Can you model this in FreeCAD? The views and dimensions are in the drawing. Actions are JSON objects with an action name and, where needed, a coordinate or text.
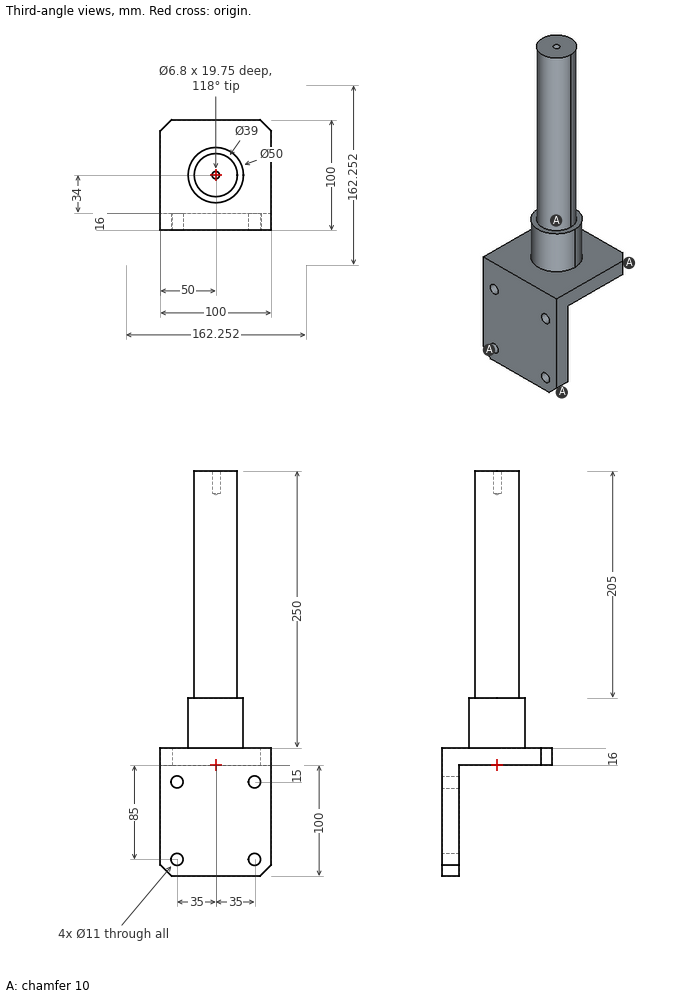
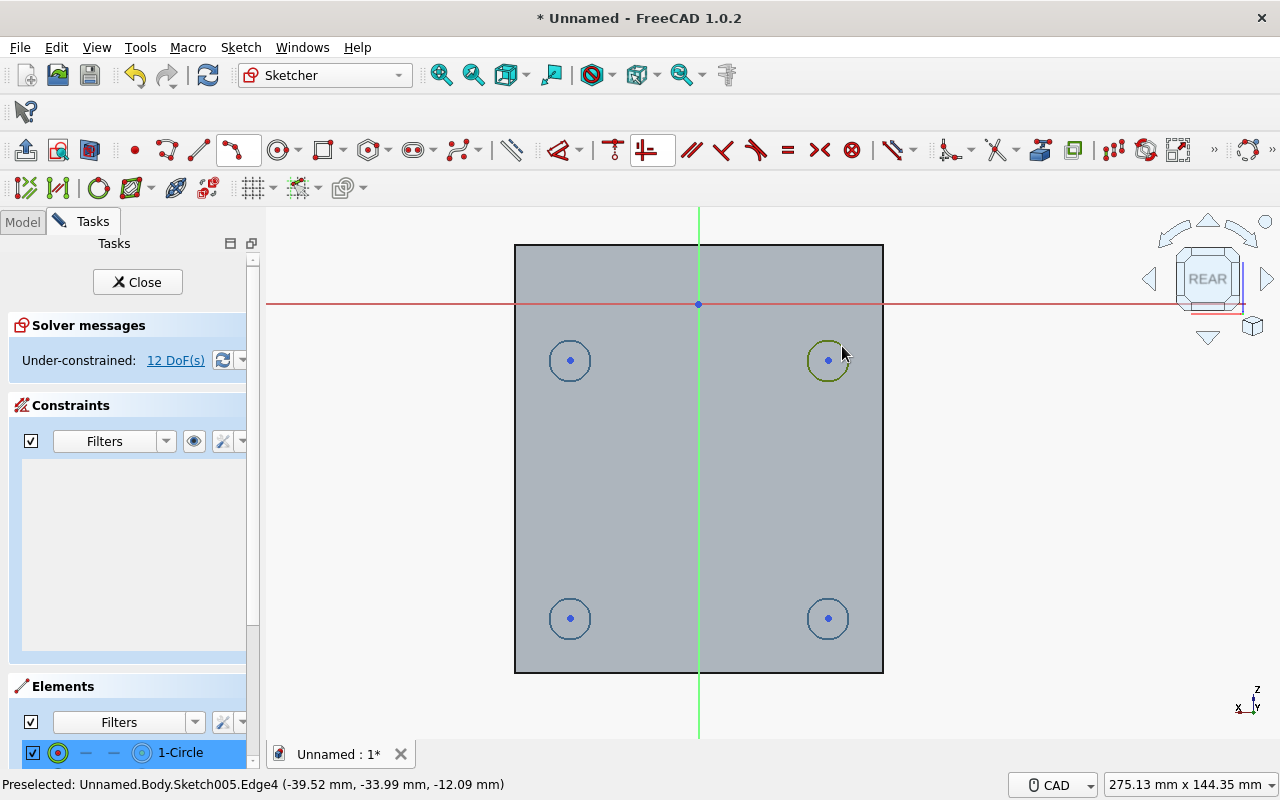
{"action": "key", "text": "e"}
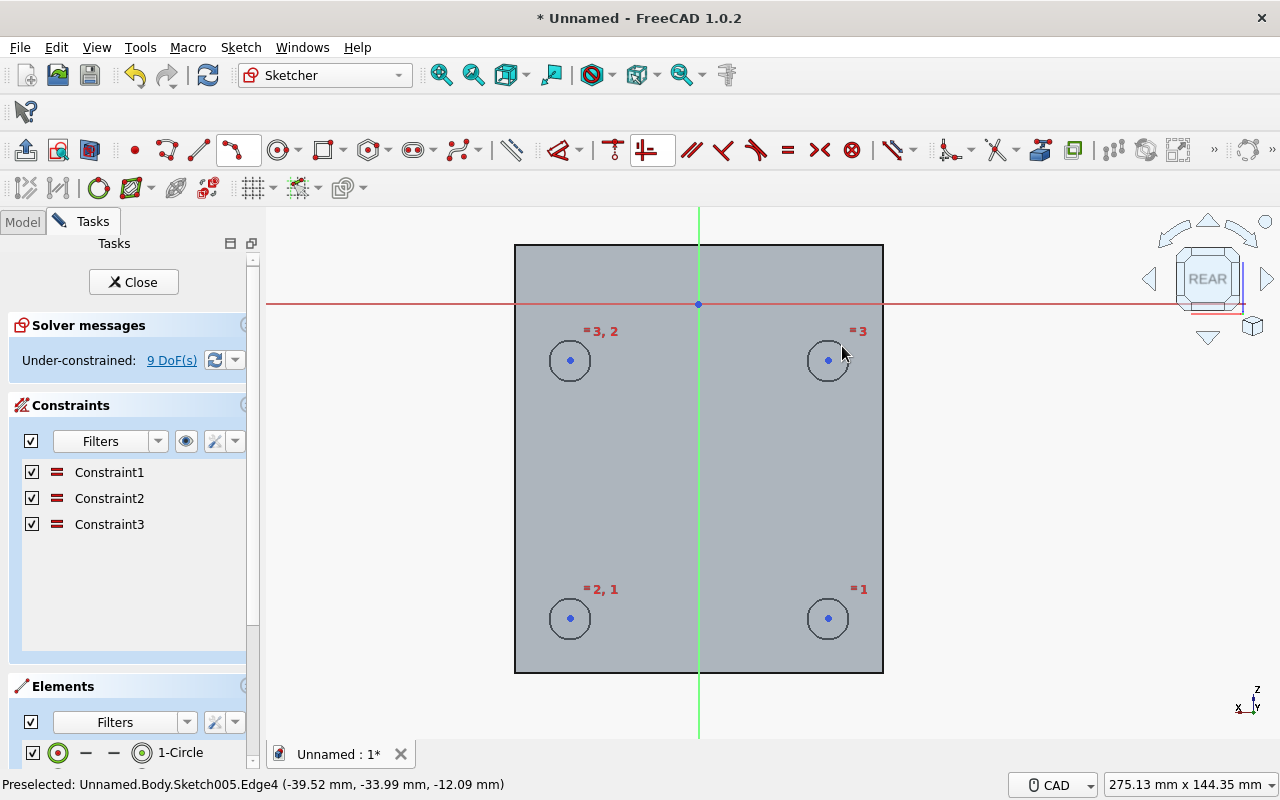
{"action": "left_click", "coordinate": [828, 619]}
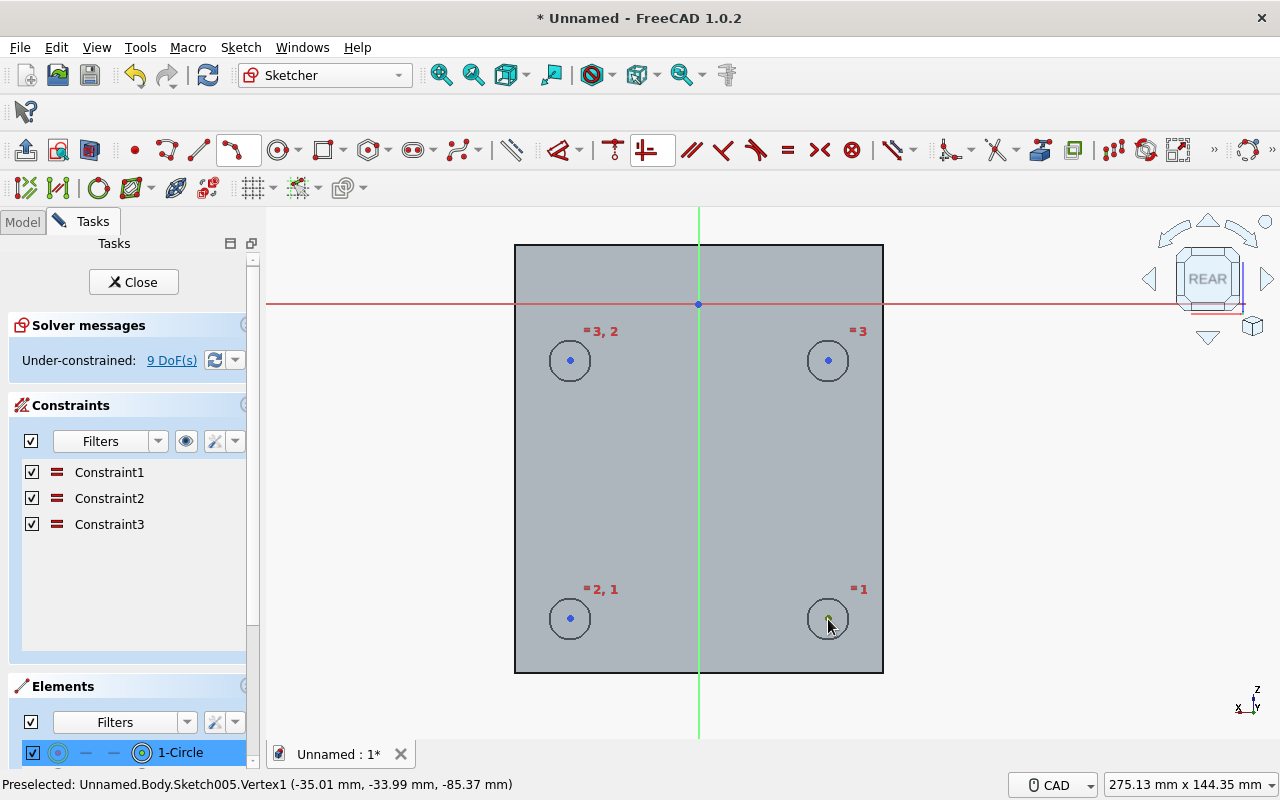
{"action": "left_click", "coordinate": [570, 619]}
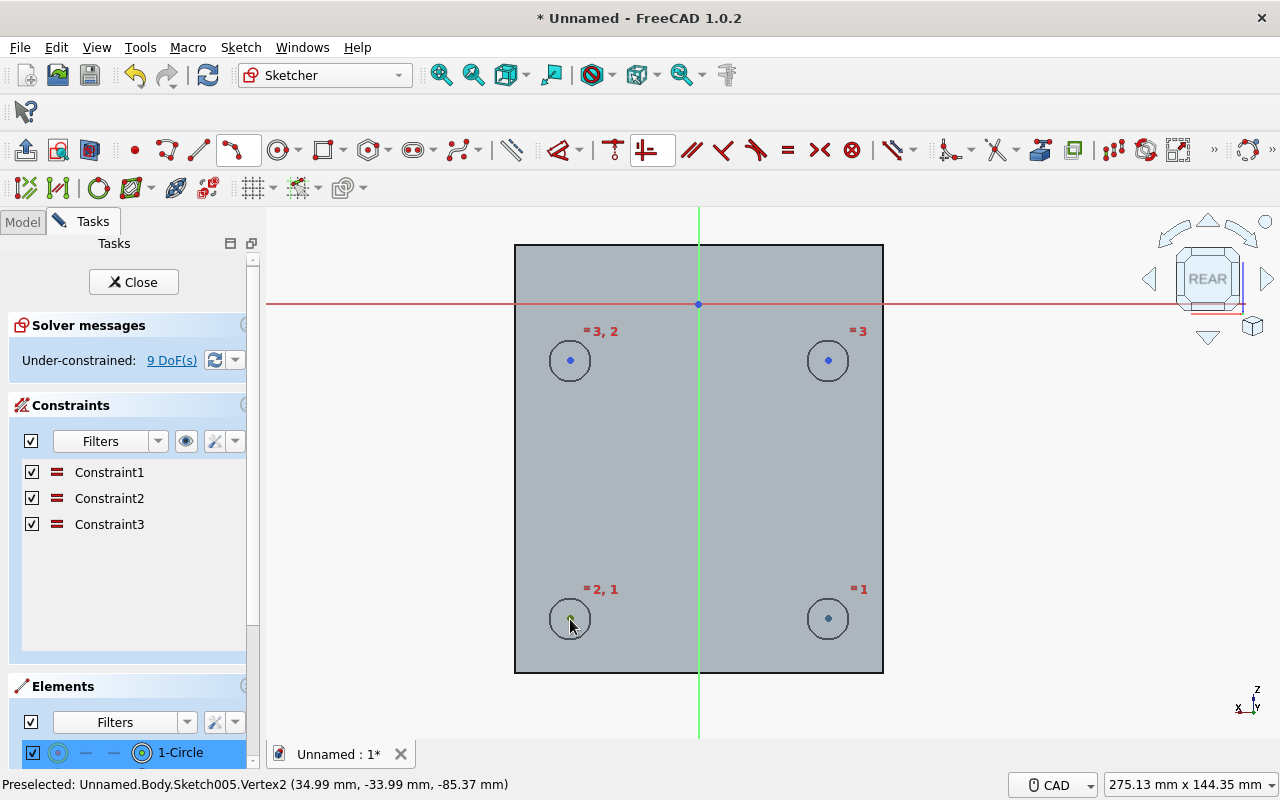
{"action": "key", "text": "h"}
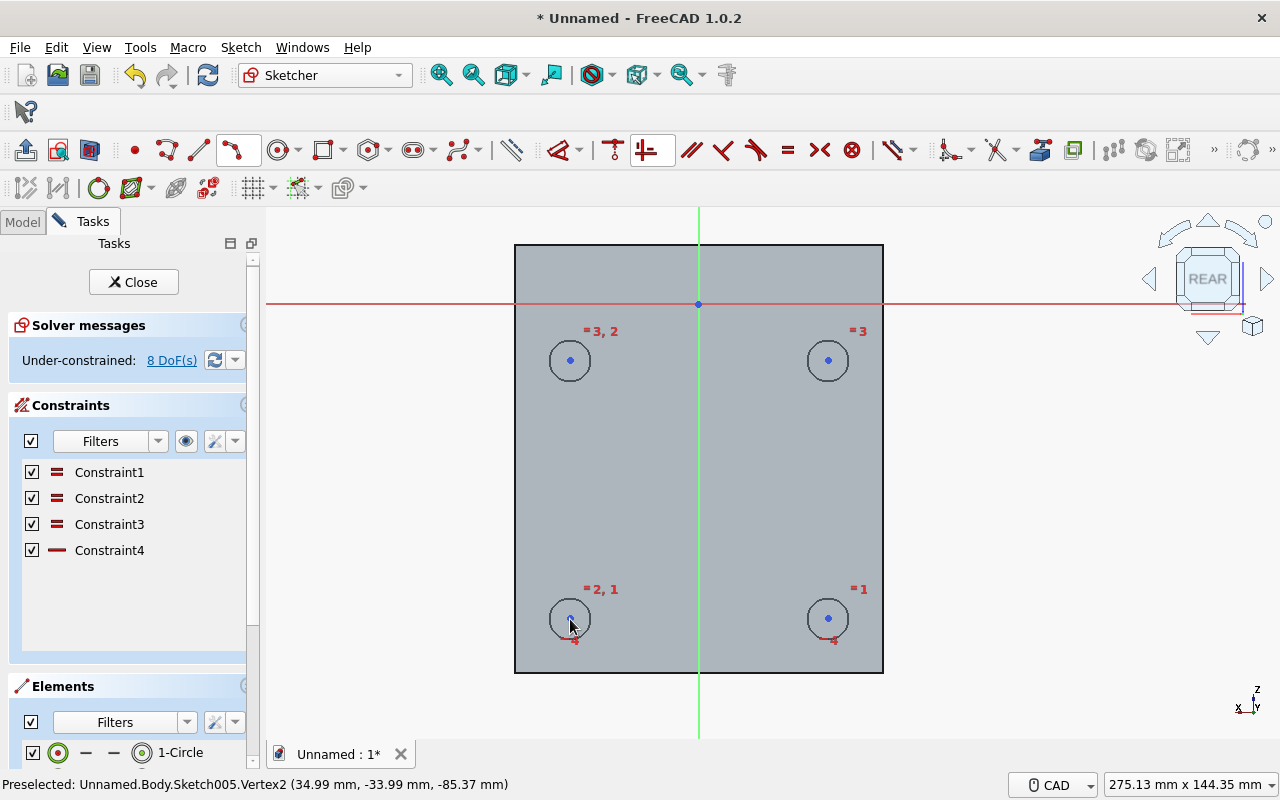
{"action": "left_click", "coordinate": [570, 619]}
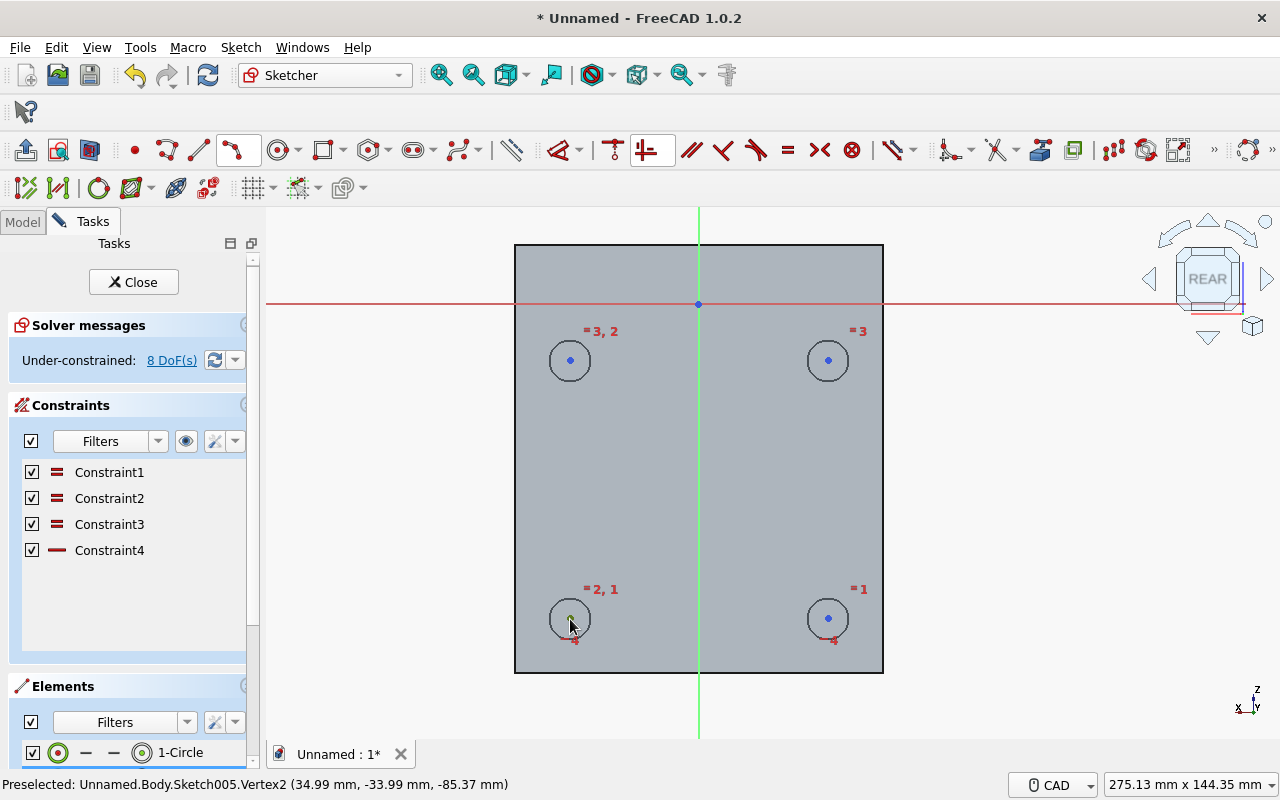
{"action": "left_click", "coordinate": [570, 361]}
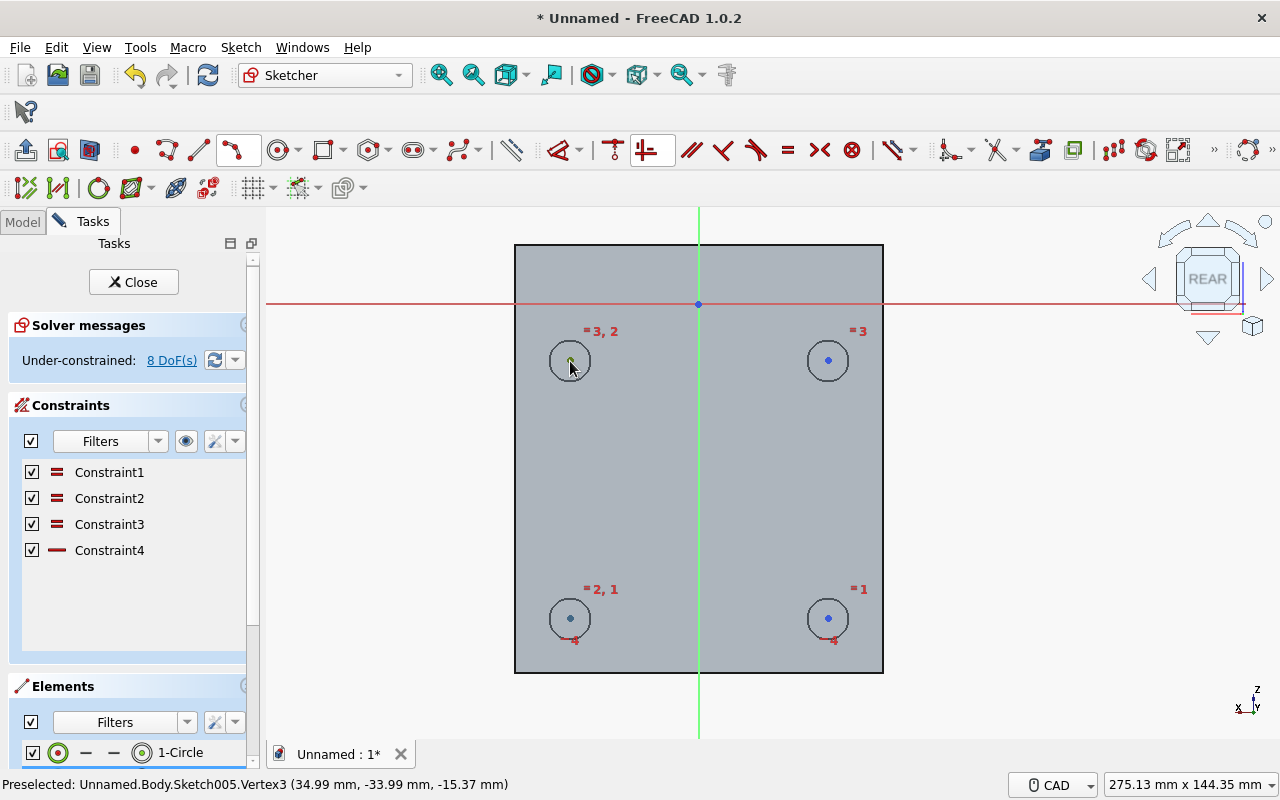
{"action": "key", "text": "v"}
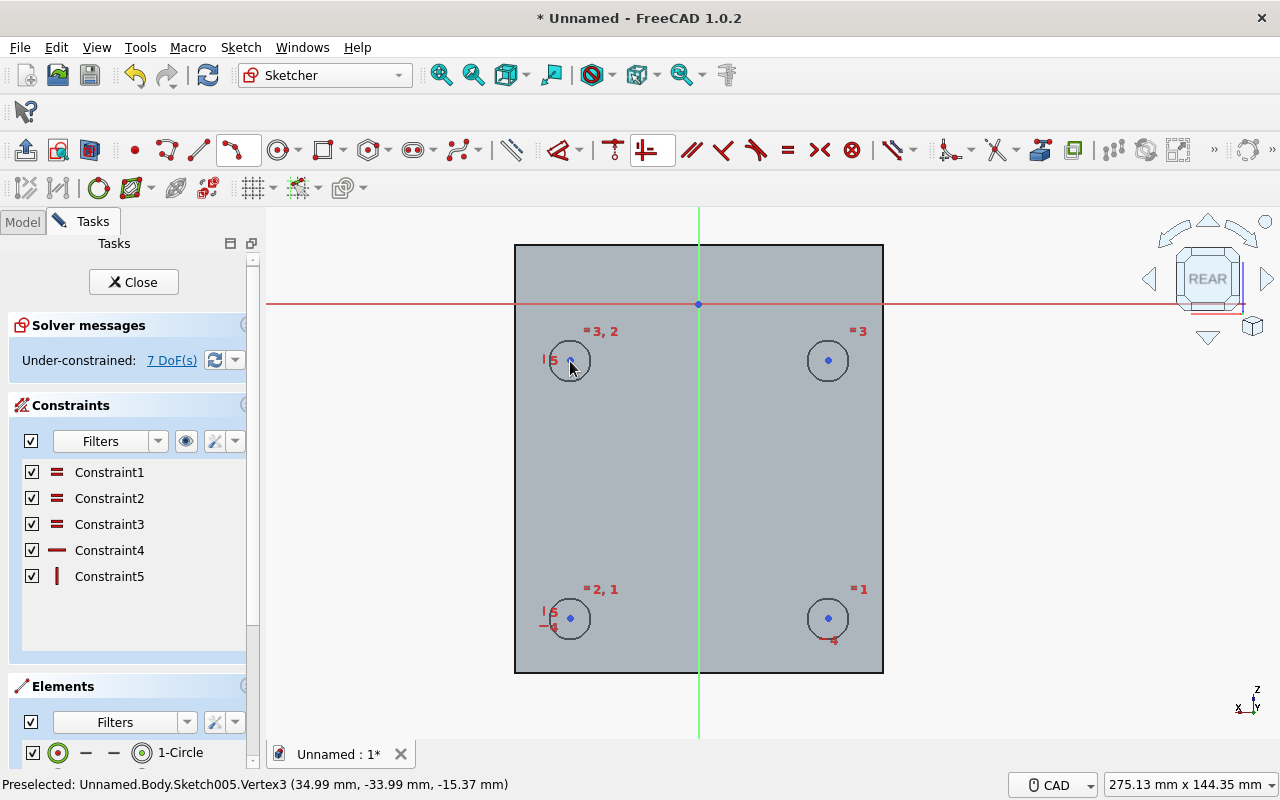
{"action": "left_click", "coordinate": [828, 619]}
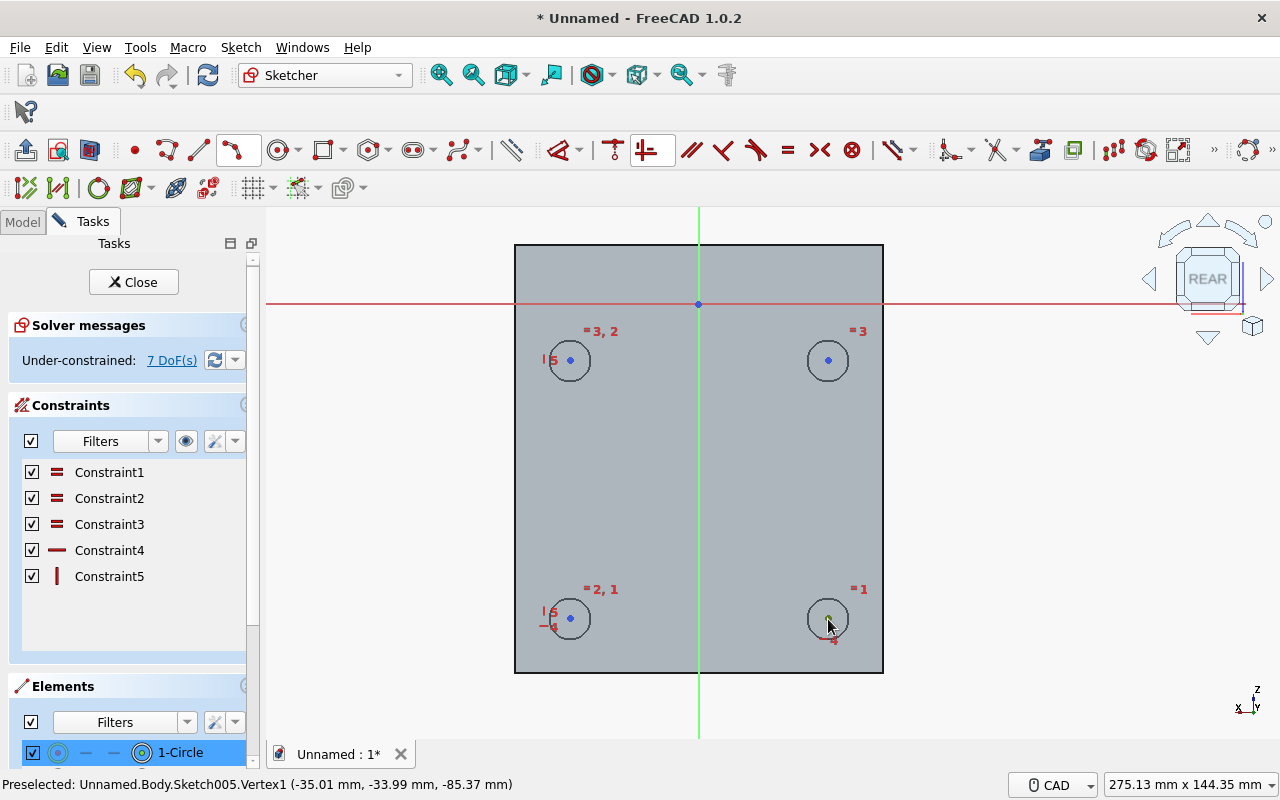
{"action": "left_click", "coordinate": [828, 361]}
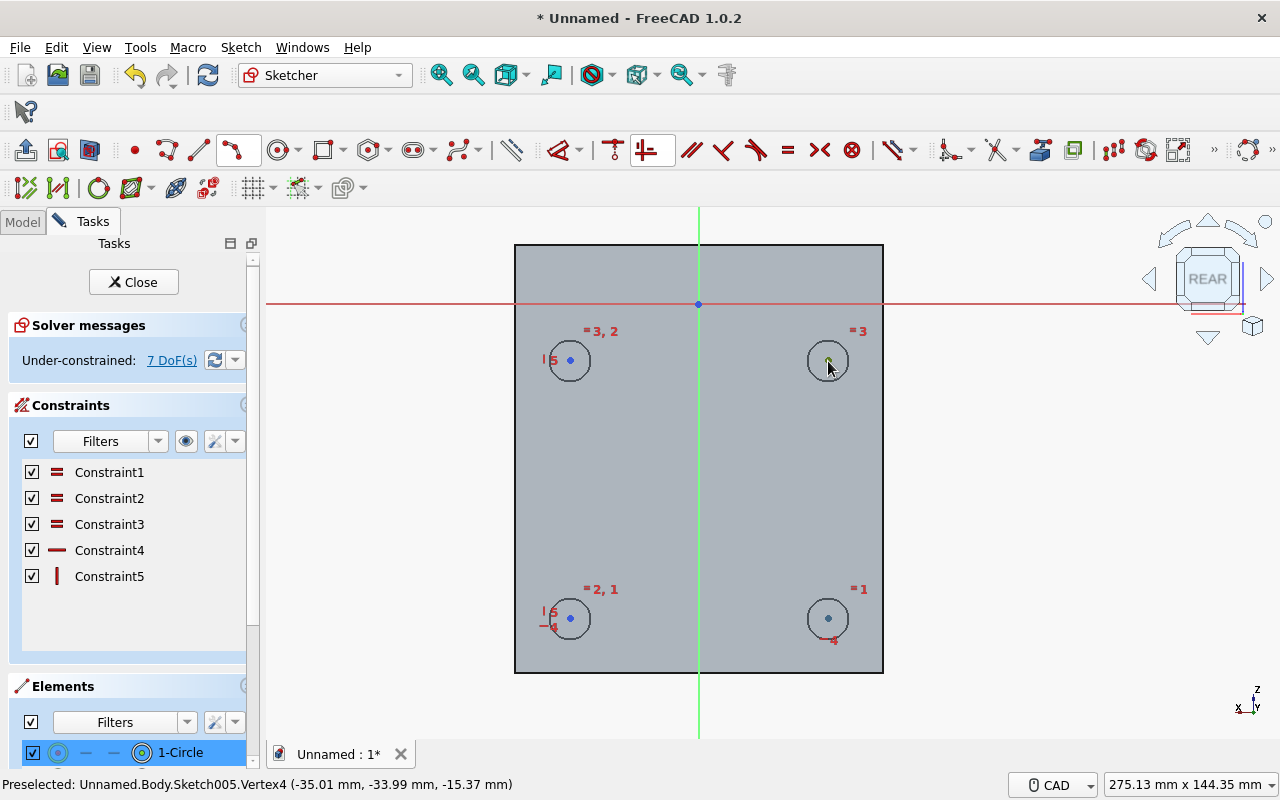
{"action": "key", "text": "v"}